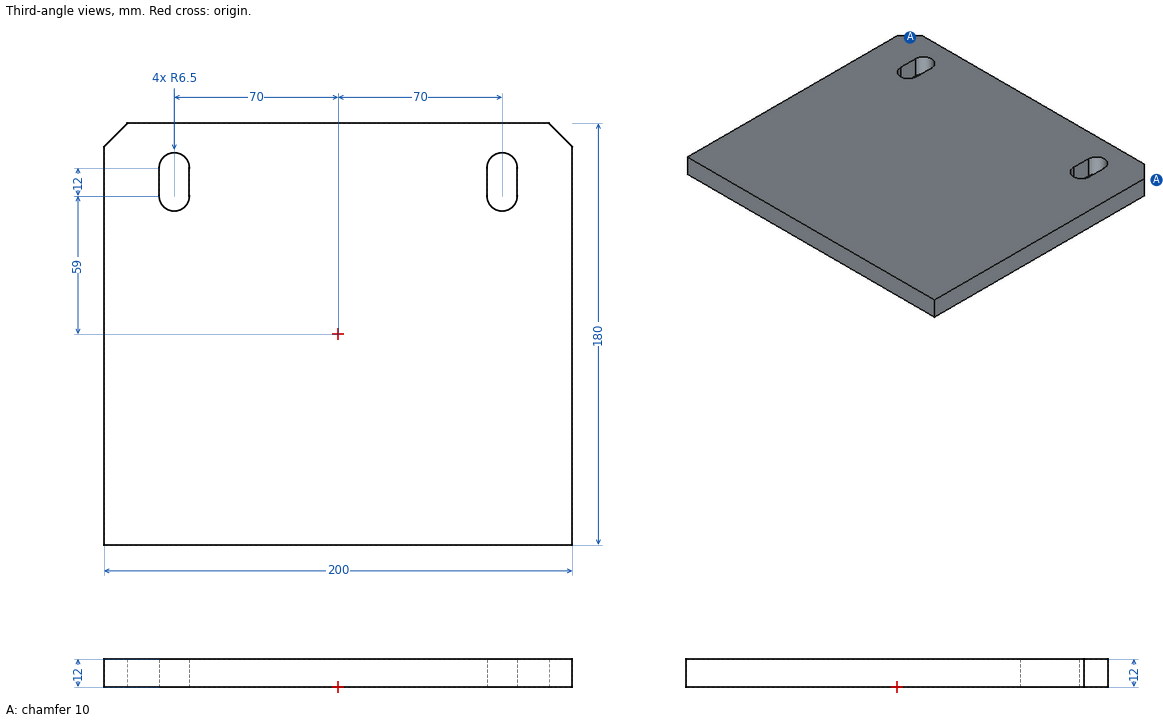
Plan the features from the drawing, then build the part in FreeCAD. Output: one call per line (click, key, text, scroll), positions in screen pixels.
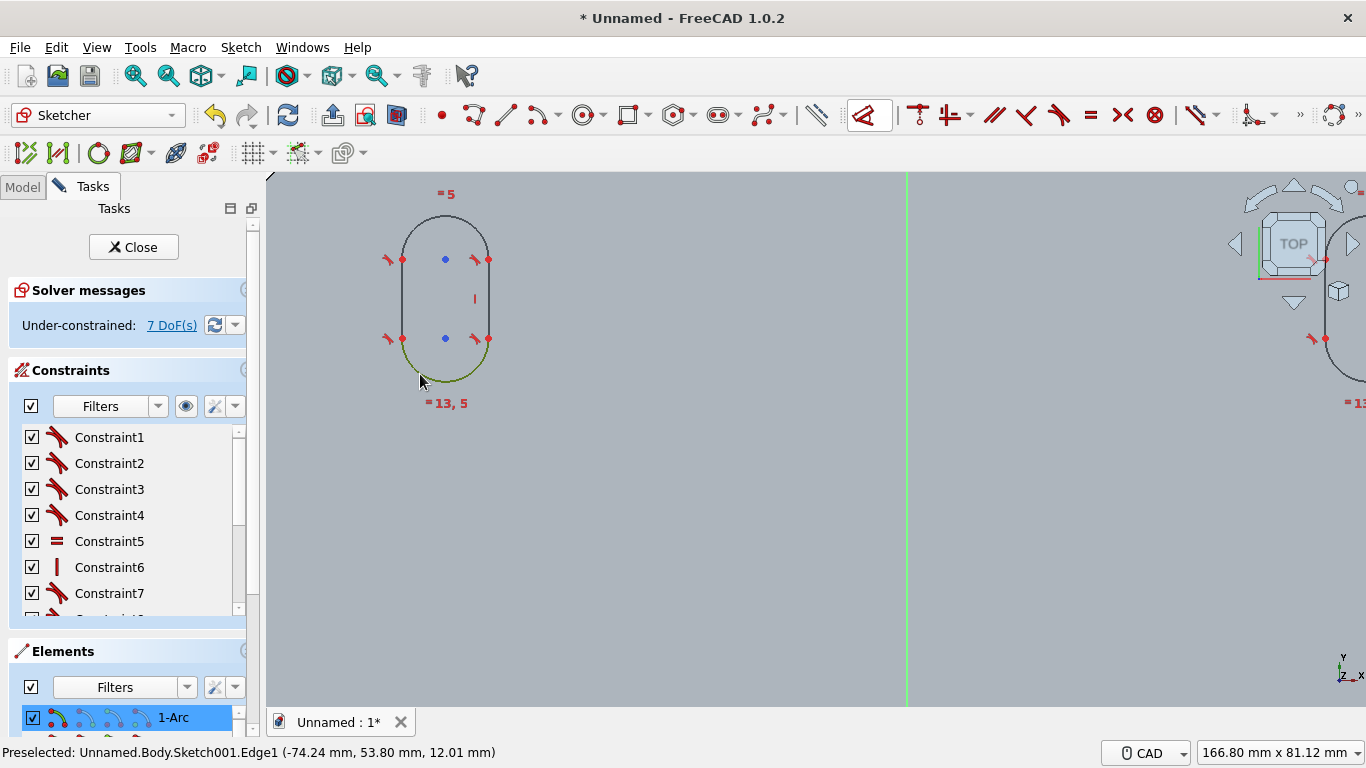
click(886, 116)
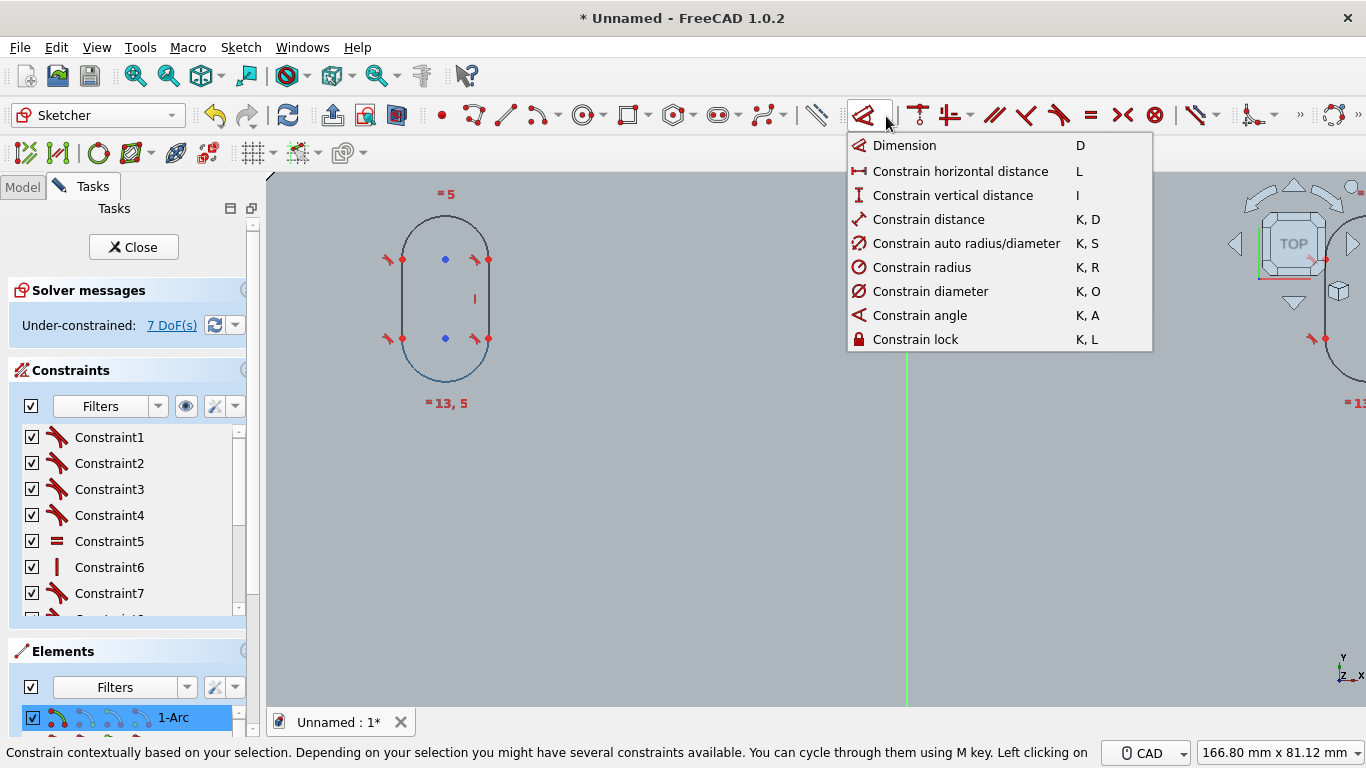
click(1000, 267)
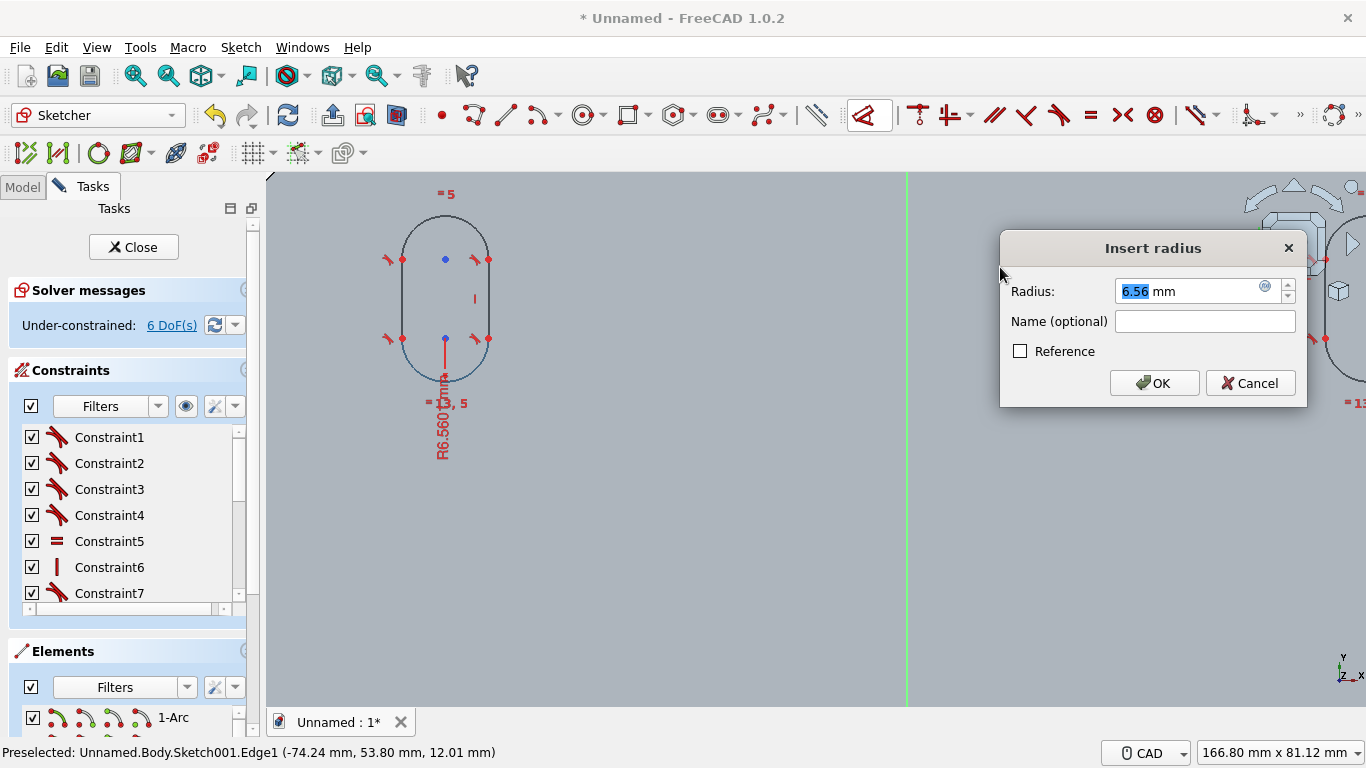
text(6.5)
key(Return)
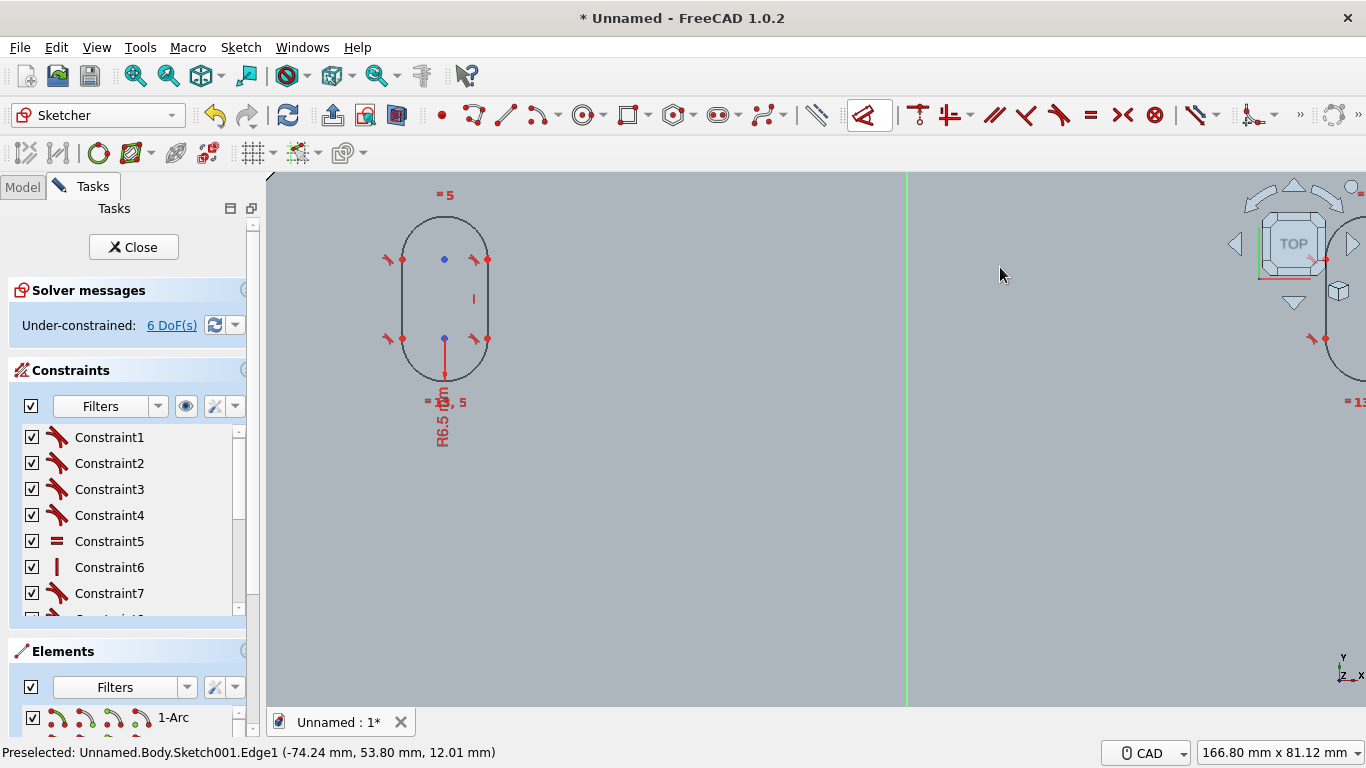
click(402, 315)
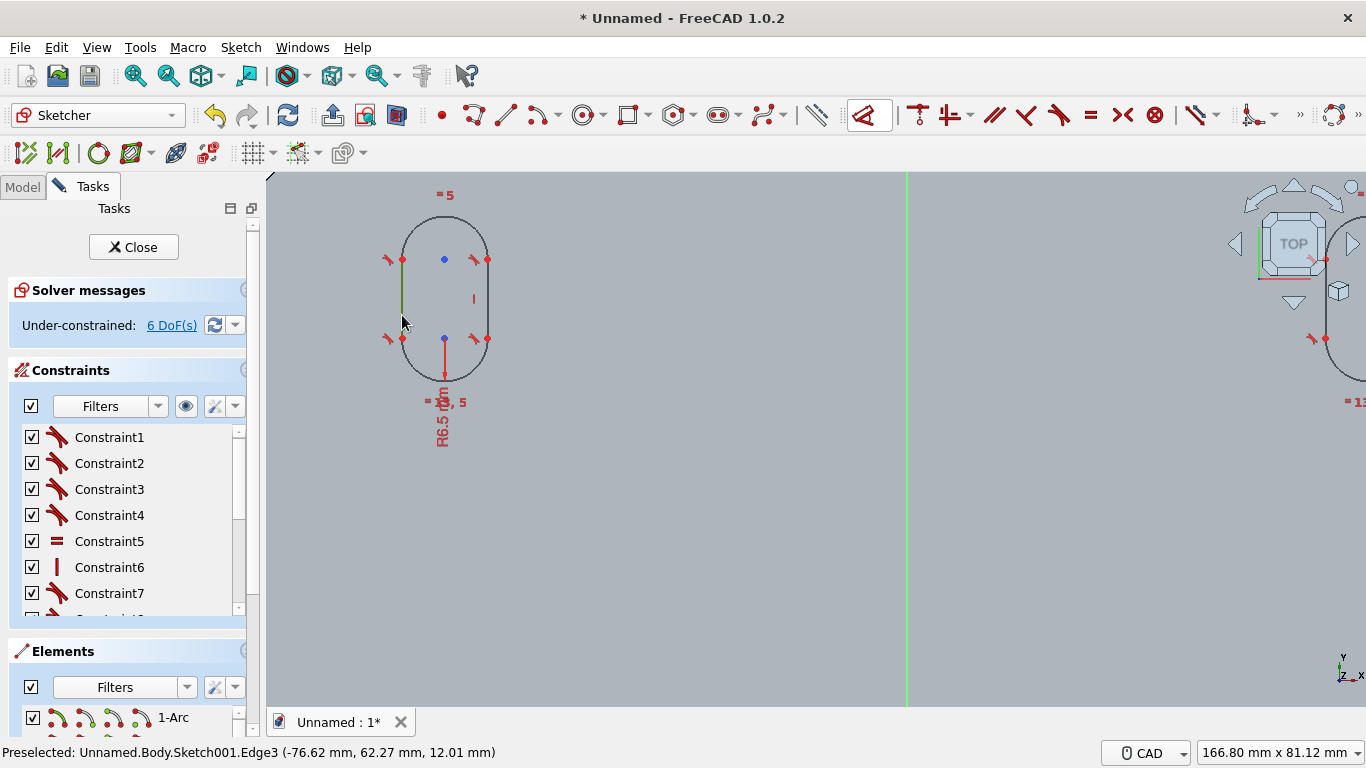
click(886, 116)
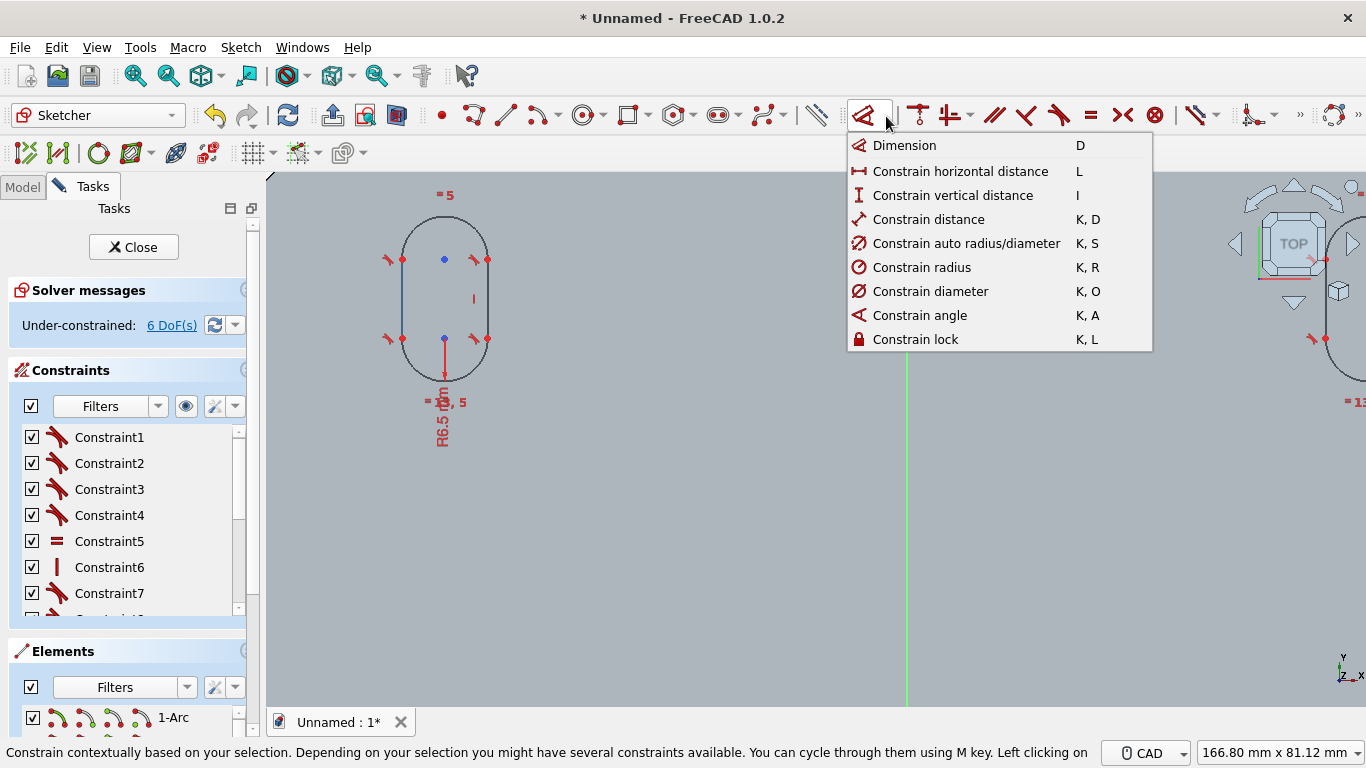
click(1000, 195)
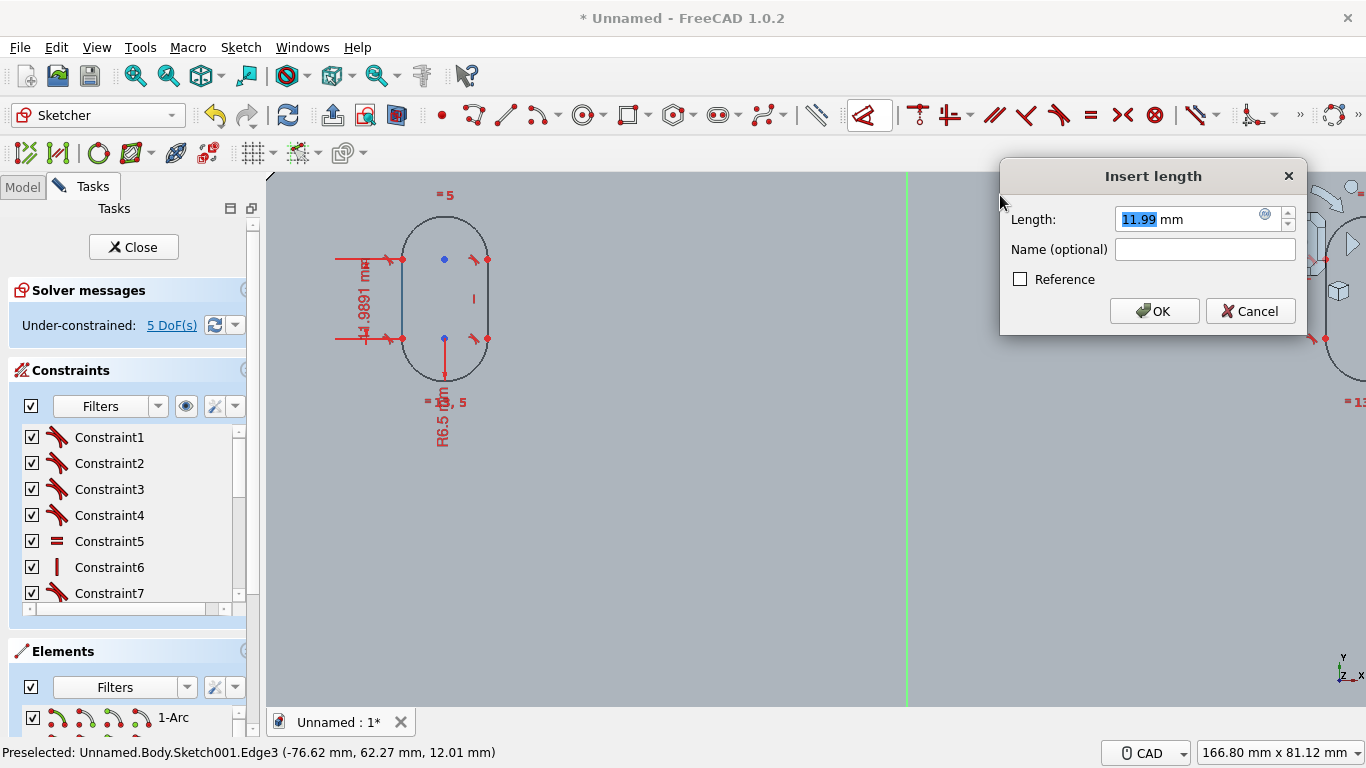
text(12)
key(Return)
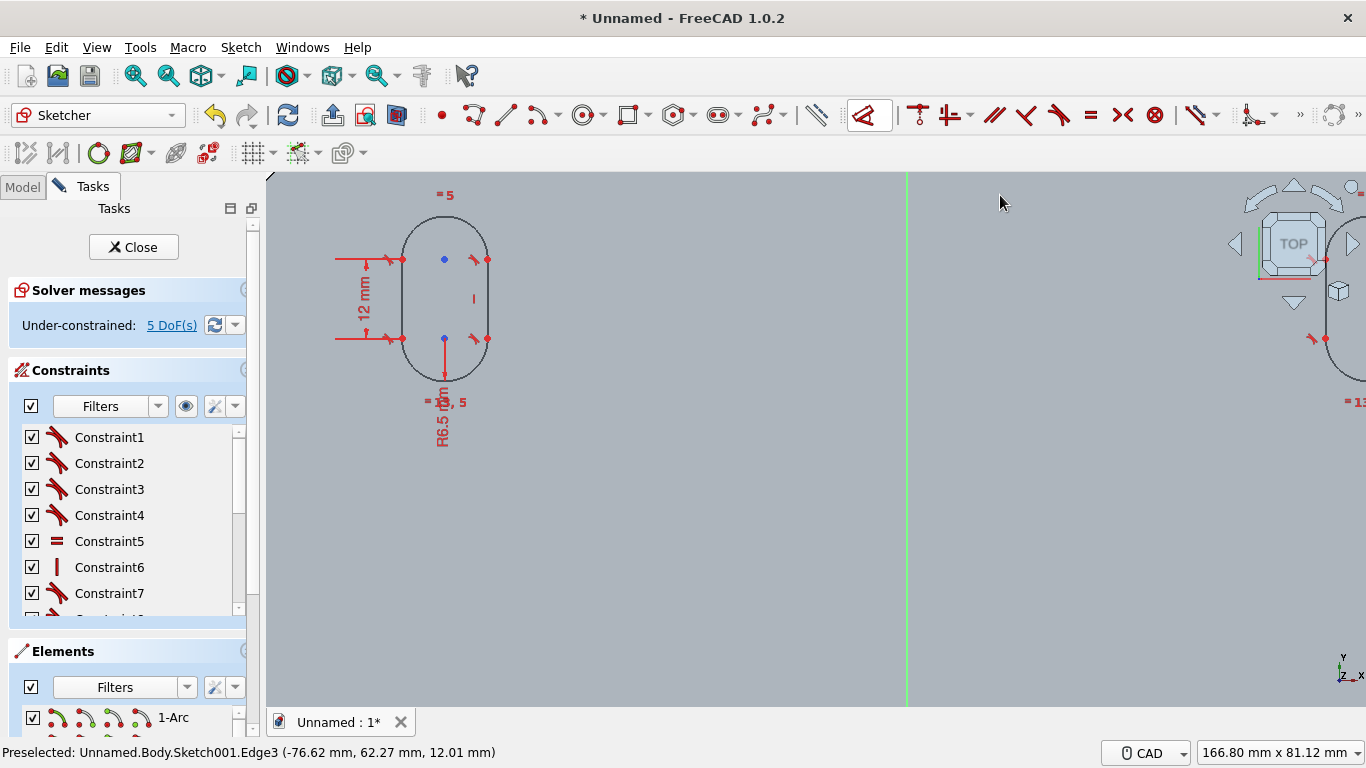
scroll(423, 375, down, 2)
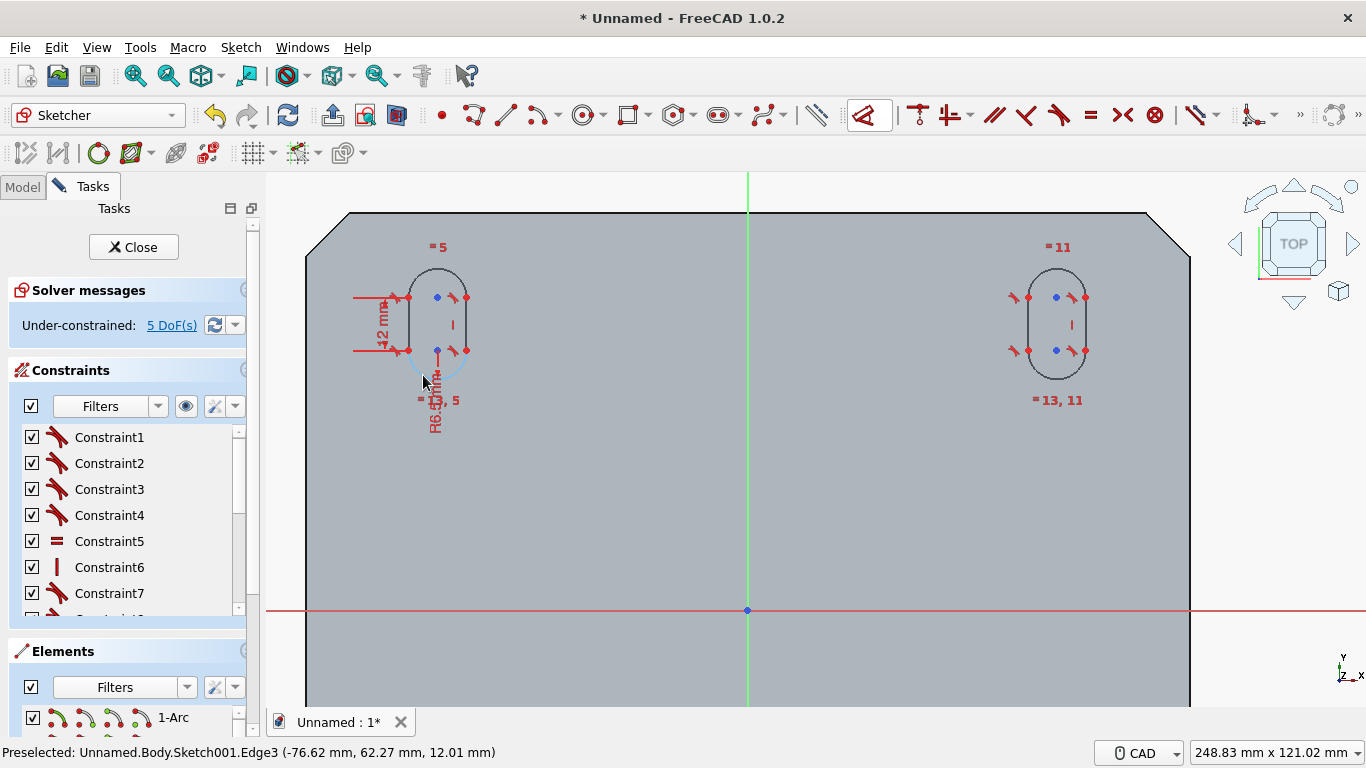
click(1028, 335)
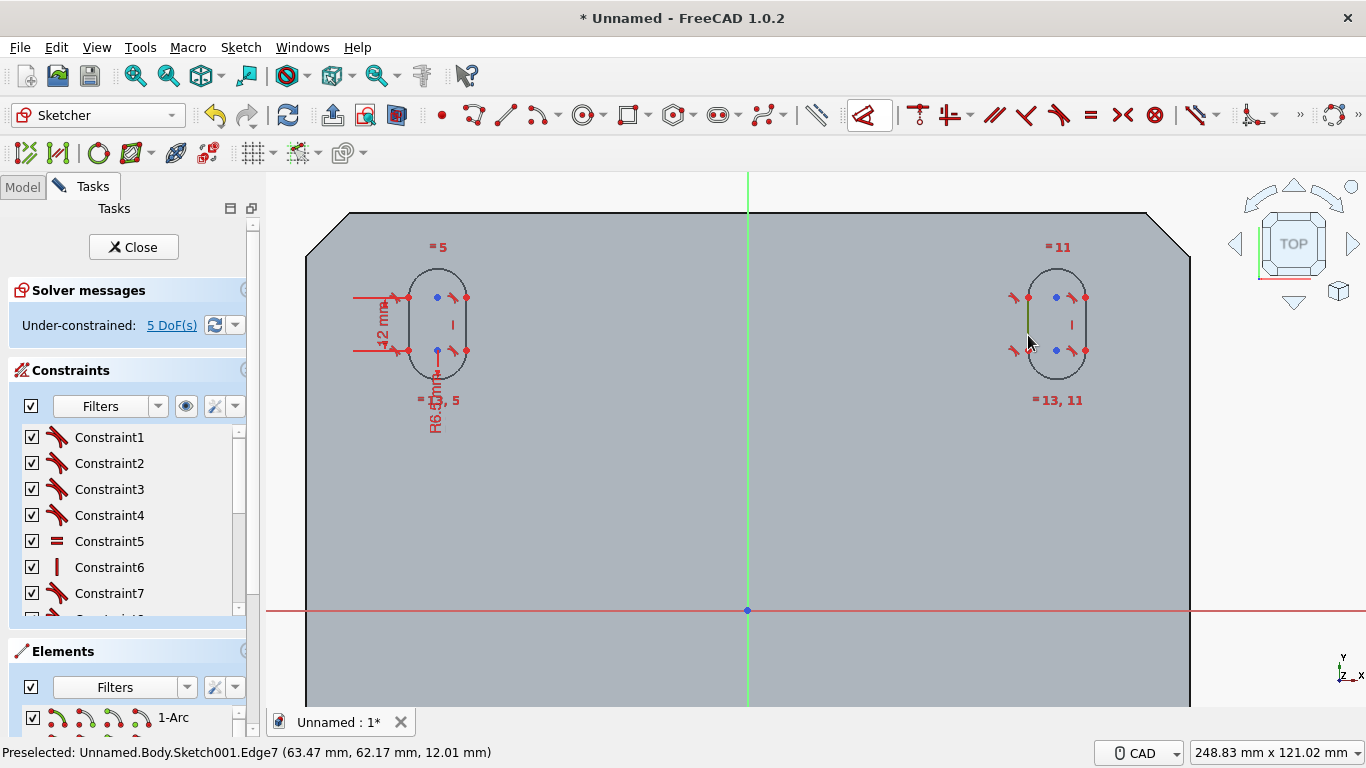
key(i)